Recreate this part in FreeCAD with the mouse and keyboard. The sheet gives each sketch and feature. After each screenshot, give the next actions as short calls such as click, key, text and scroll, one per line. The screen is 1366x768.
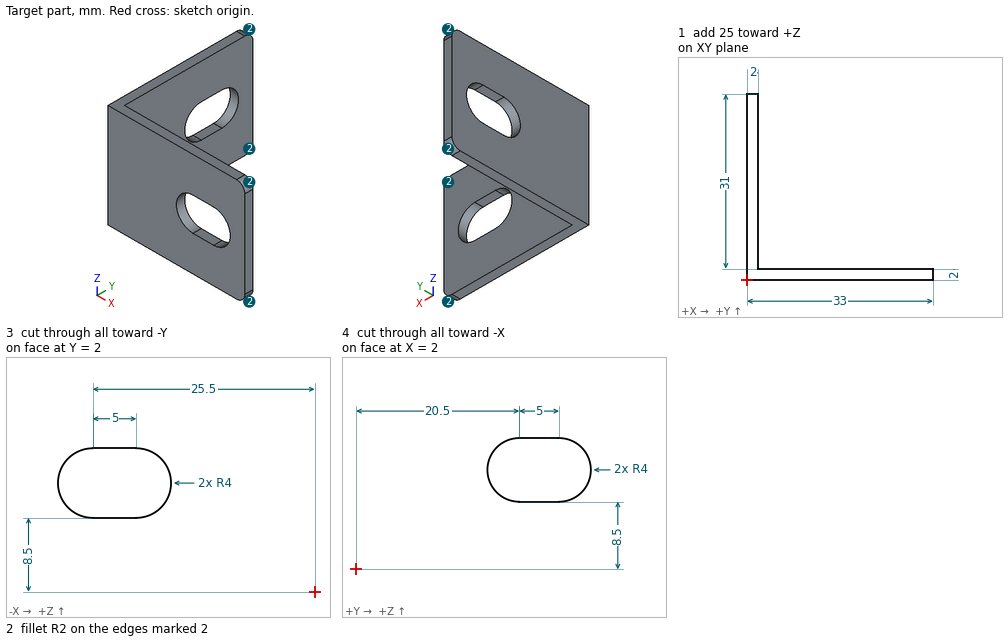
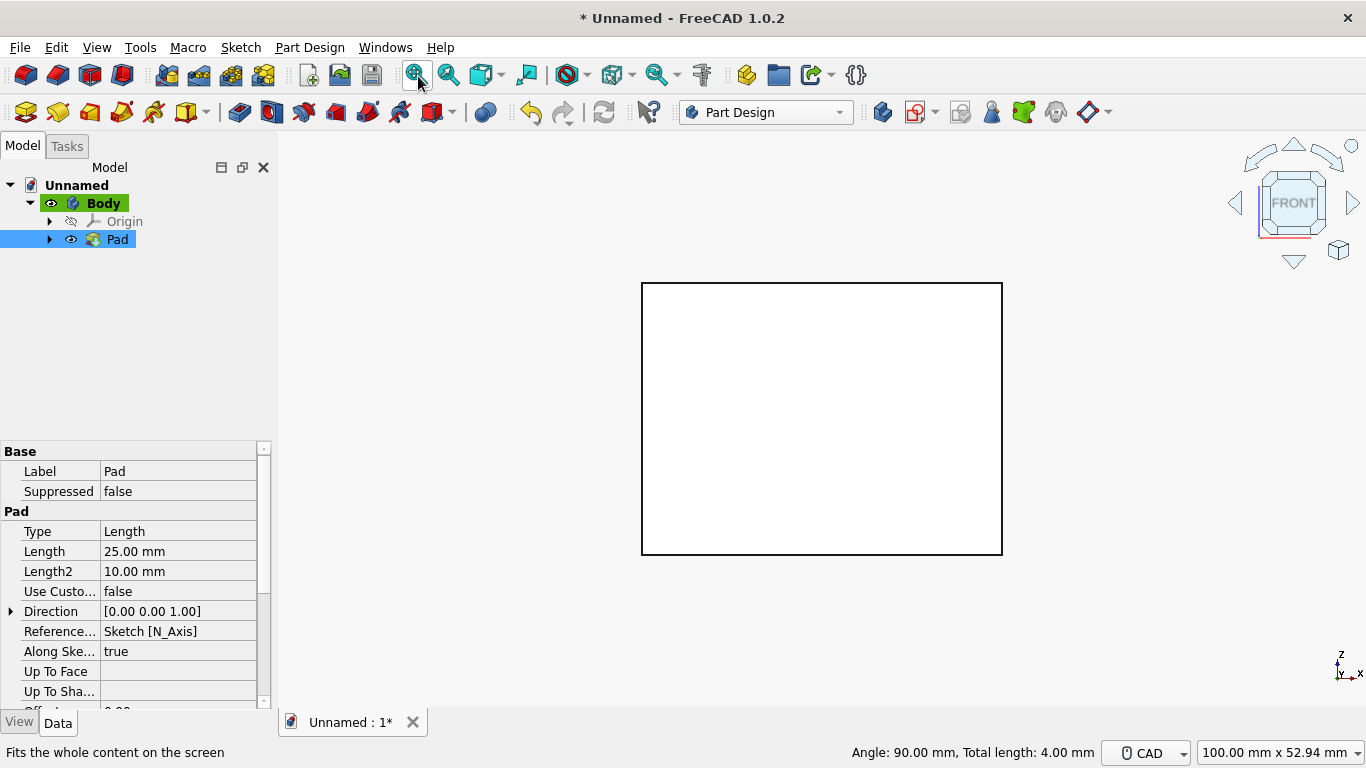
key(3)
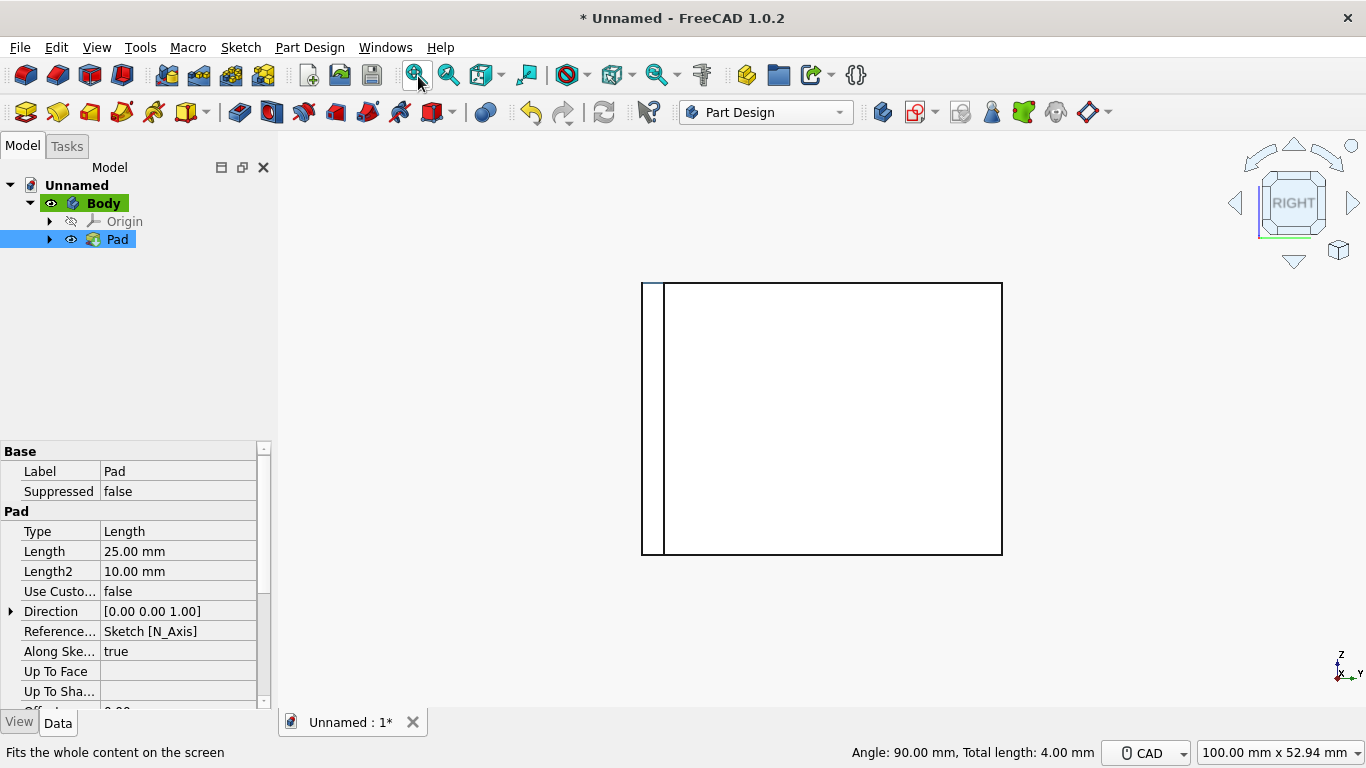
click(653, 554, ctrl)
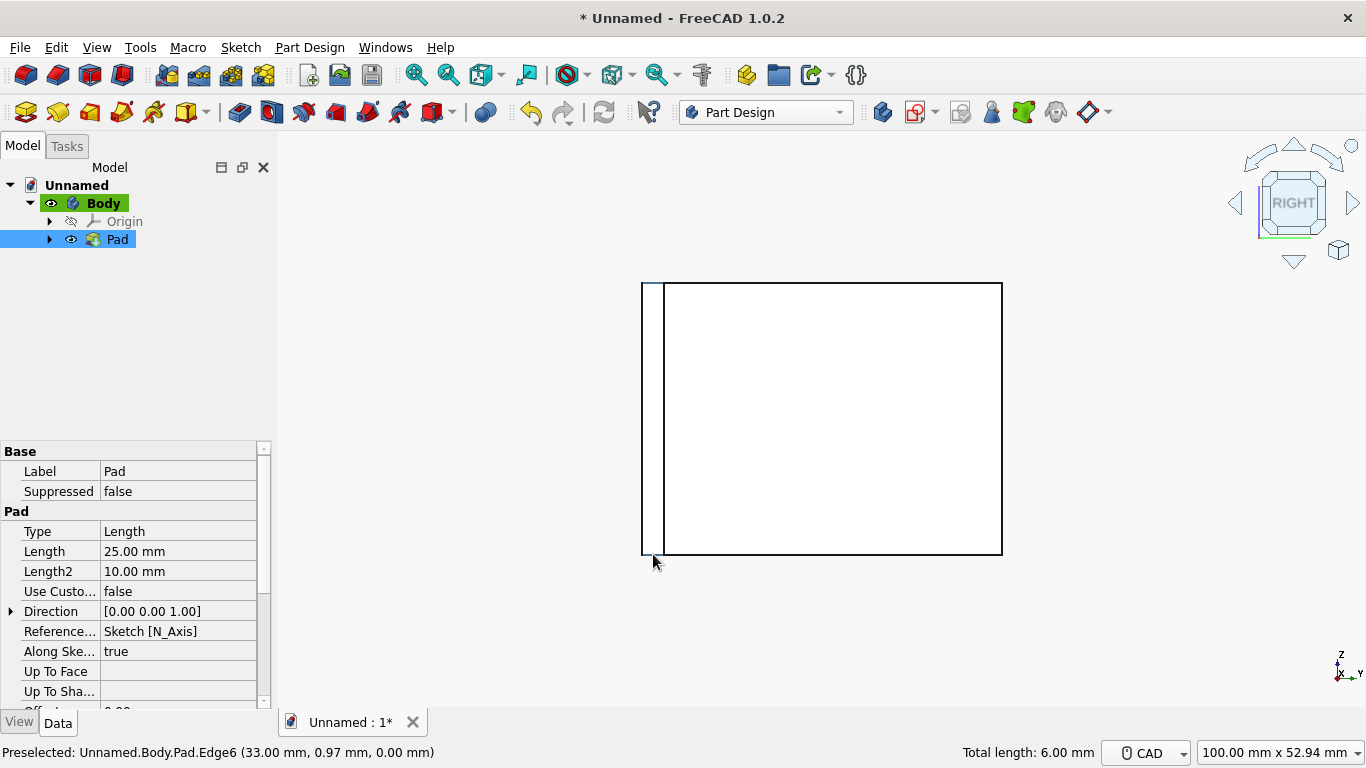
scroll(1002, 554, up, 4)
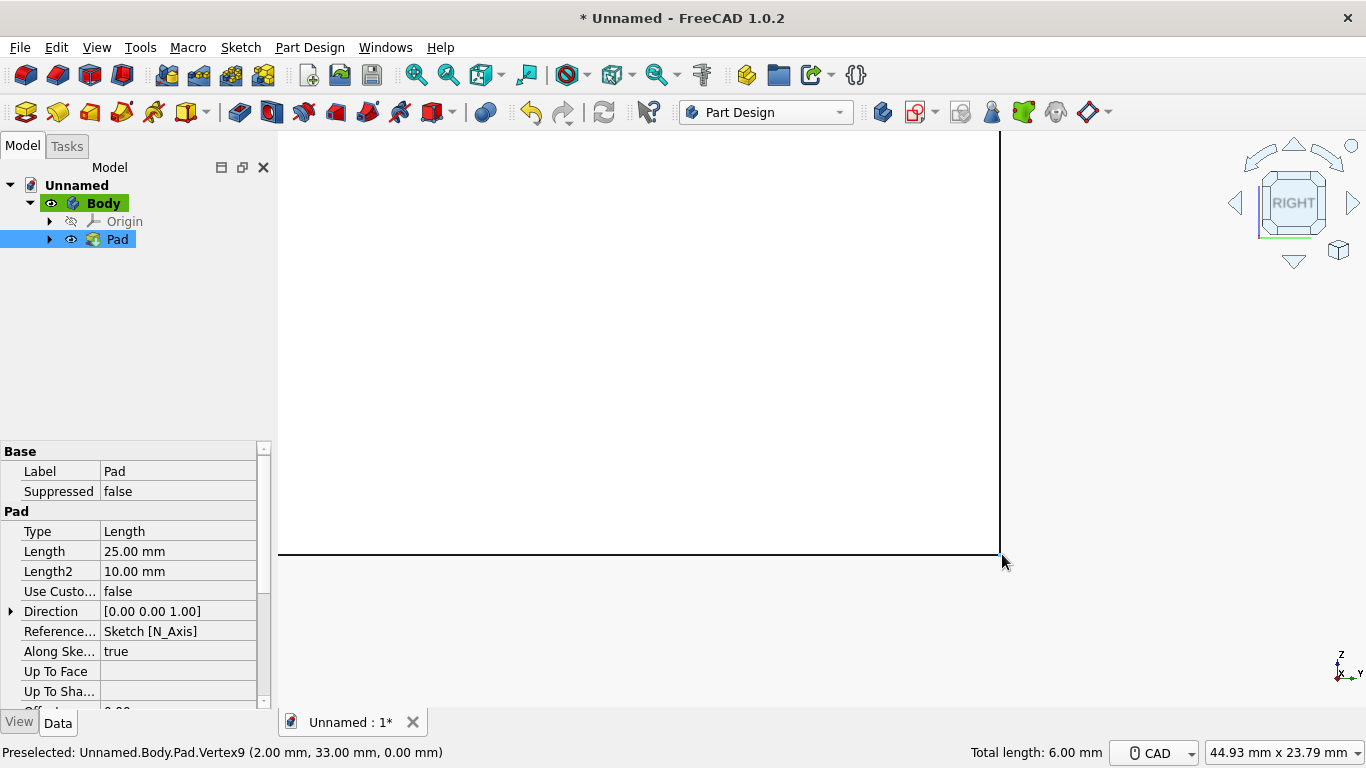
key(v)
key(f)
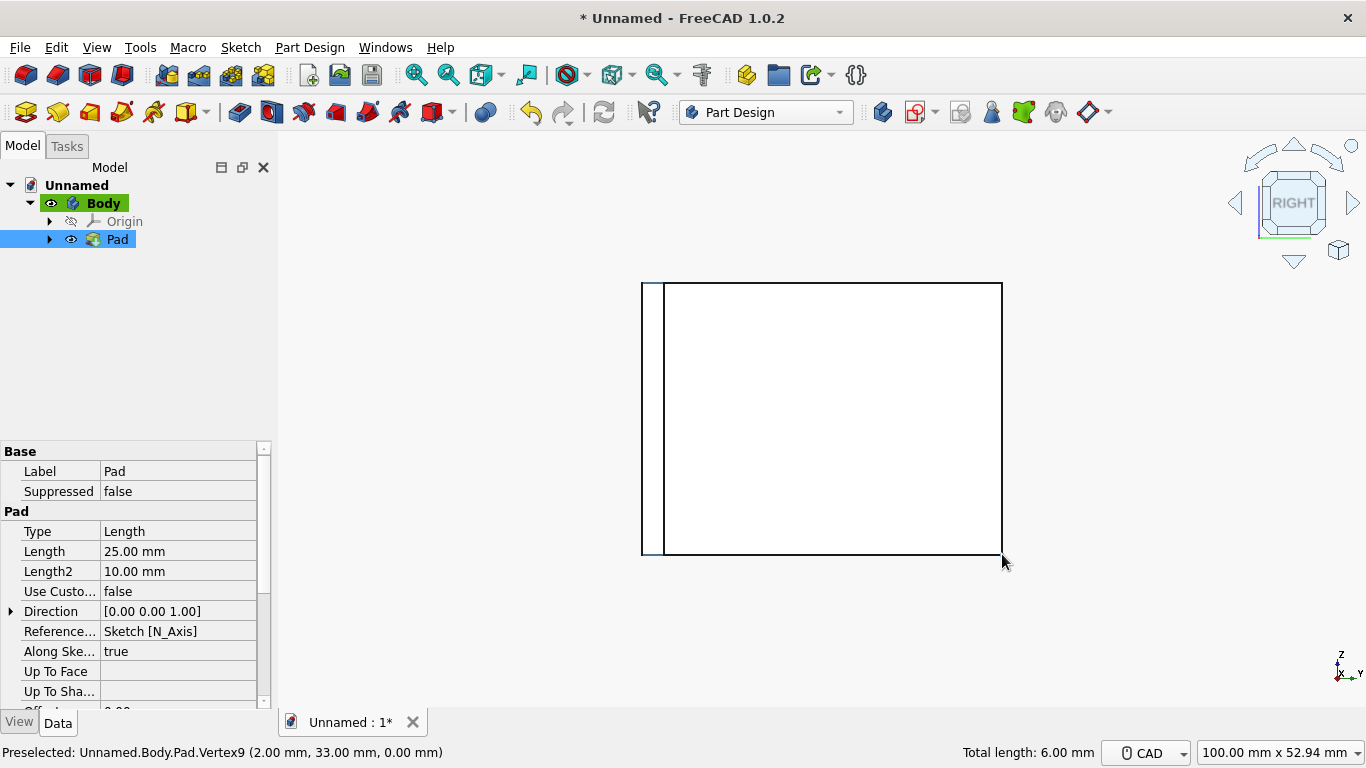
key(5)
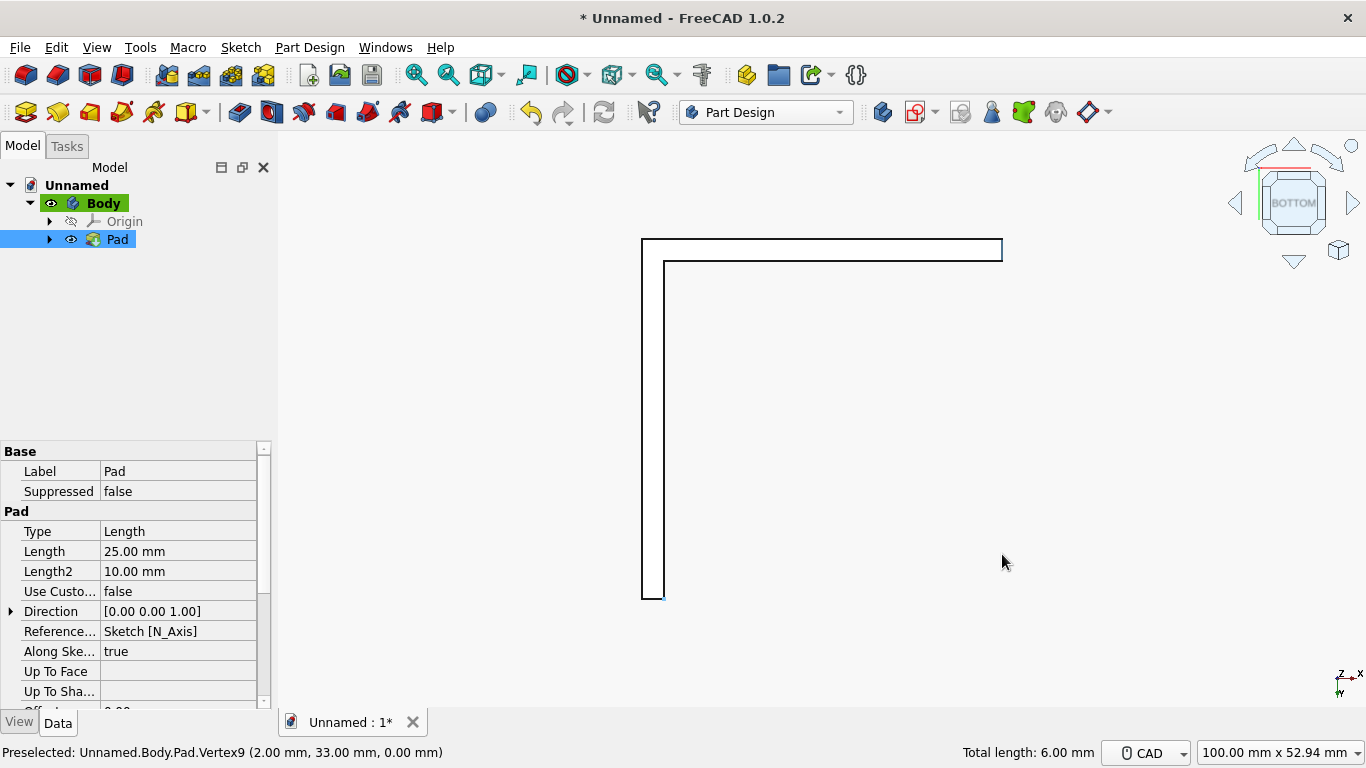
click(653, 598, ctrl)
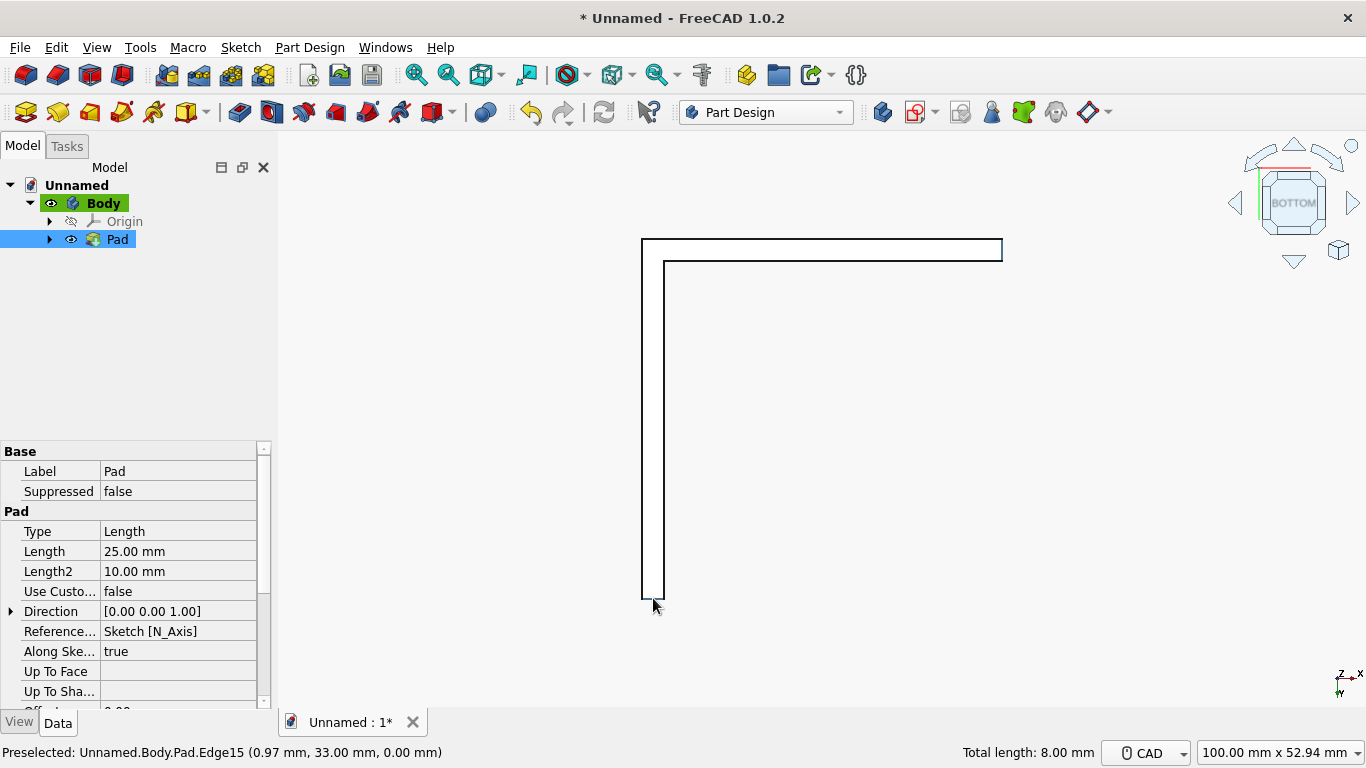
click(26, 76)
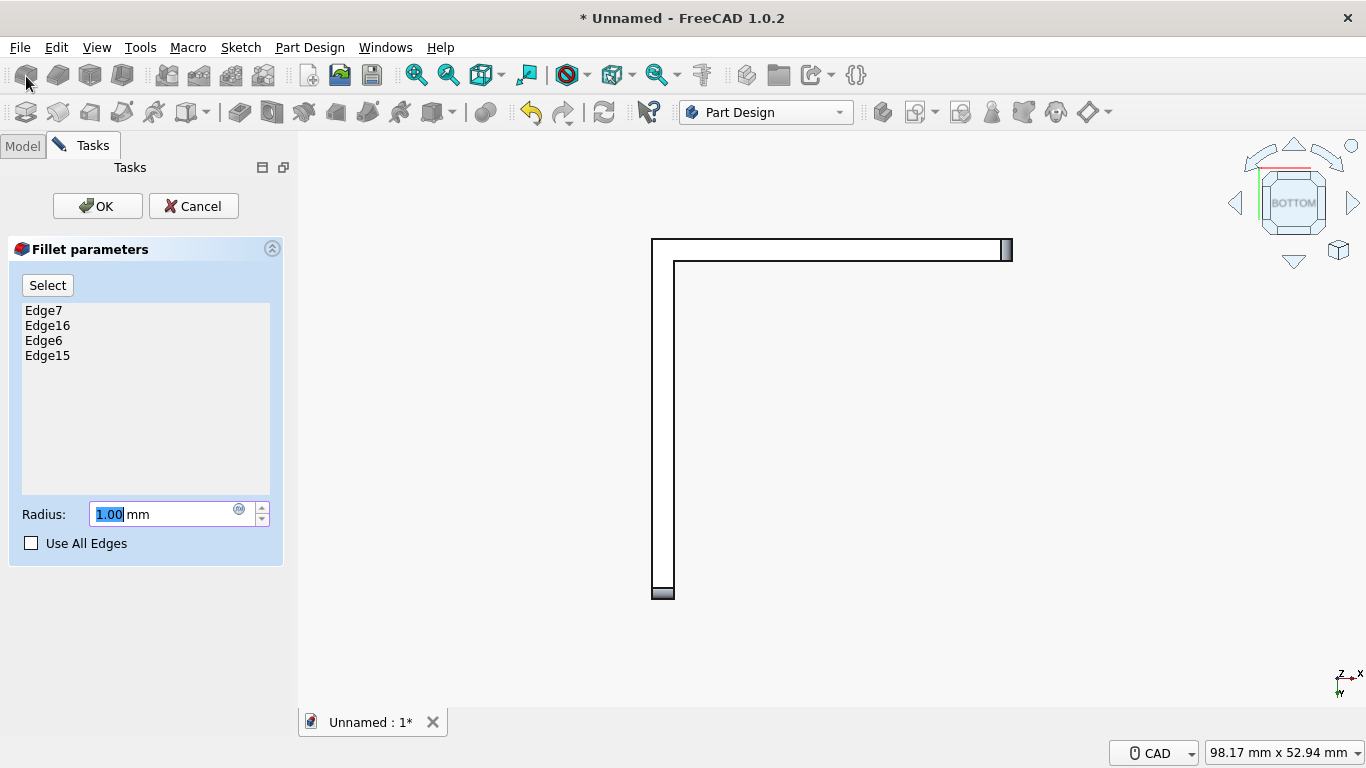
text(2)
key(Tab)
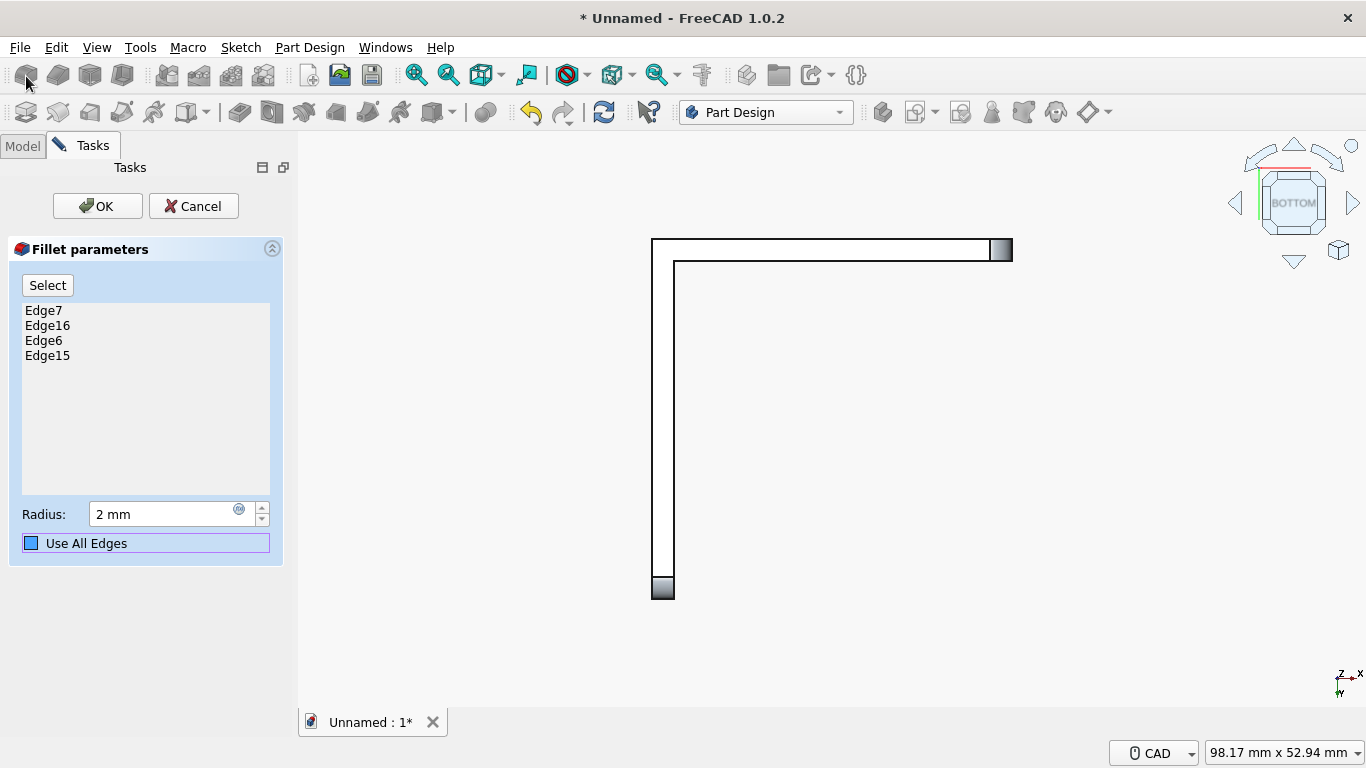
click(98, 206)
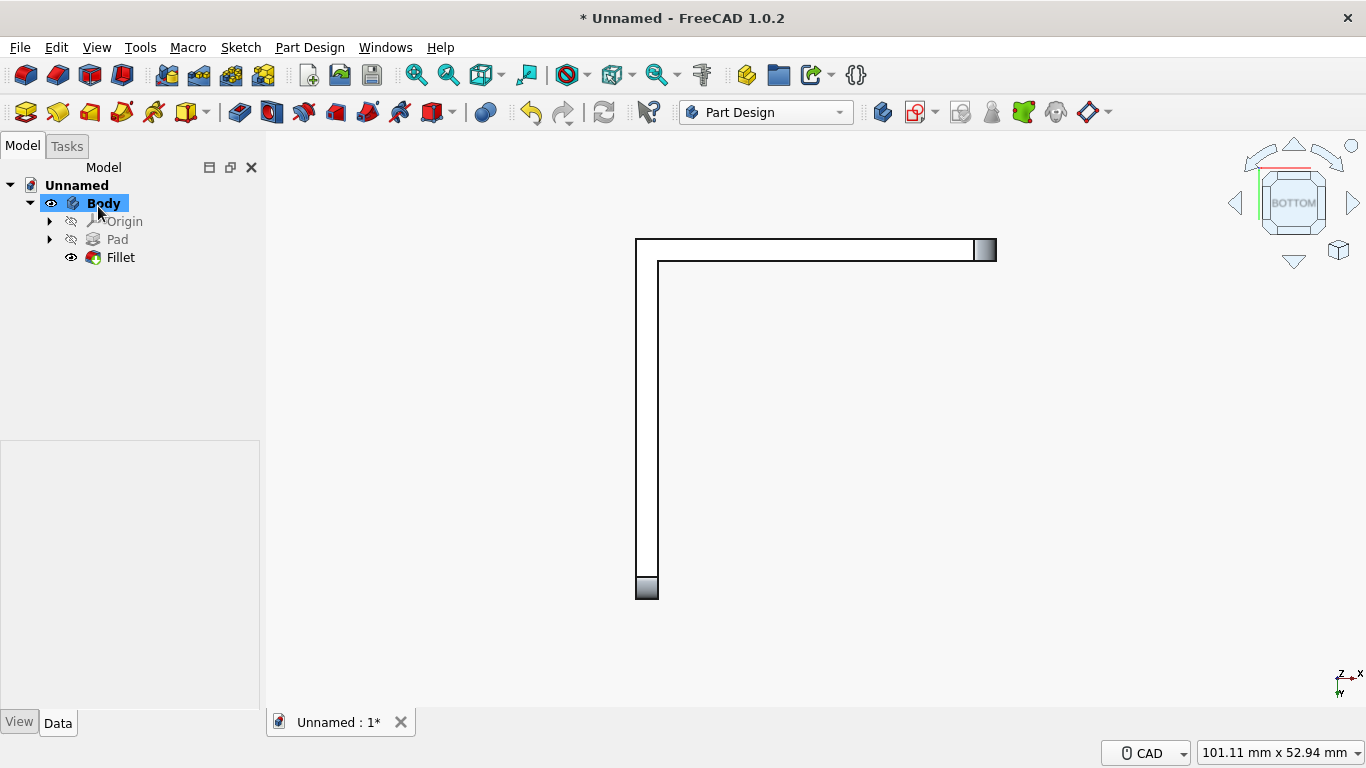
key(4)